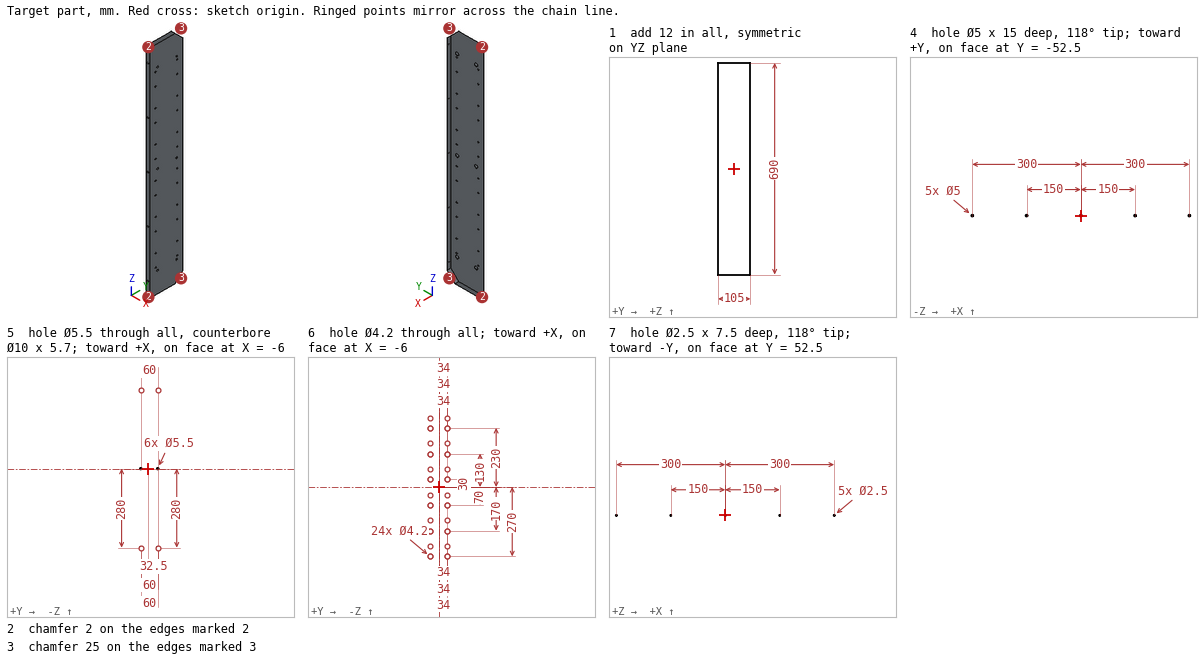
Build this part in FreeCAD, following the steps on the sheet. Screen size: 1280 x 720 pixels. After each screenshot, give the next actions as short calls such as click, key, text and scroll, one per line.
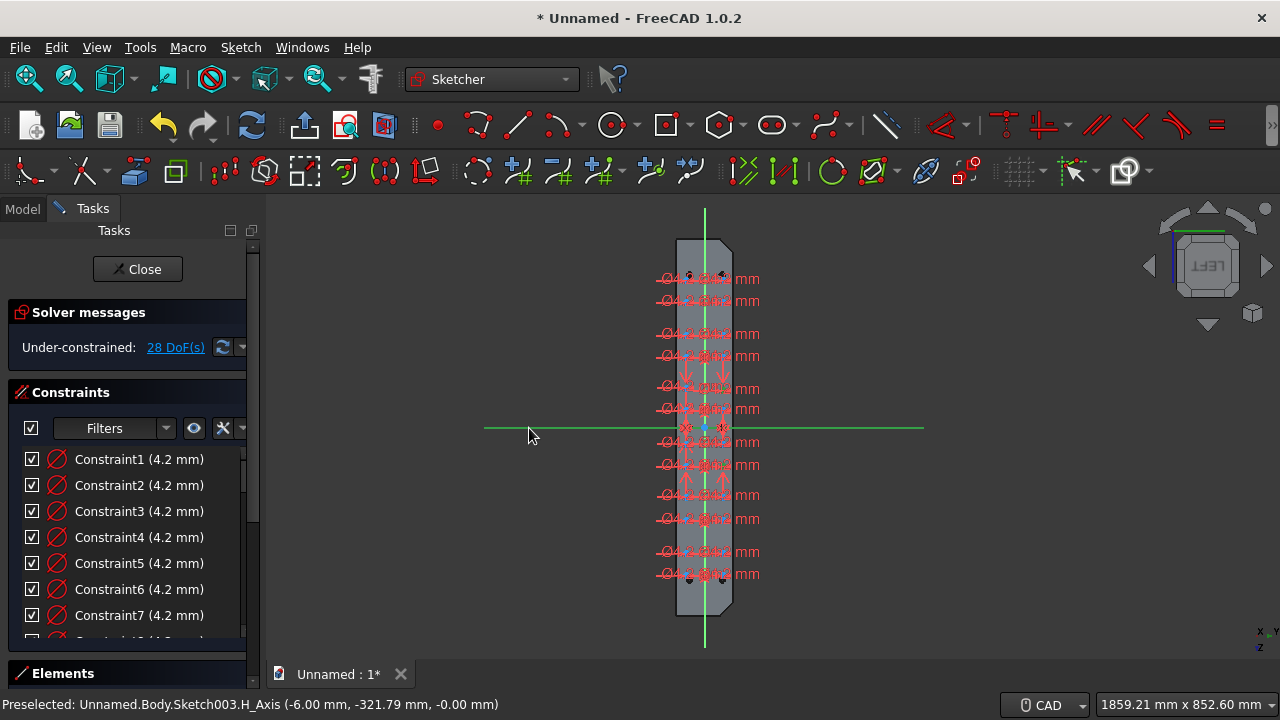
key(s)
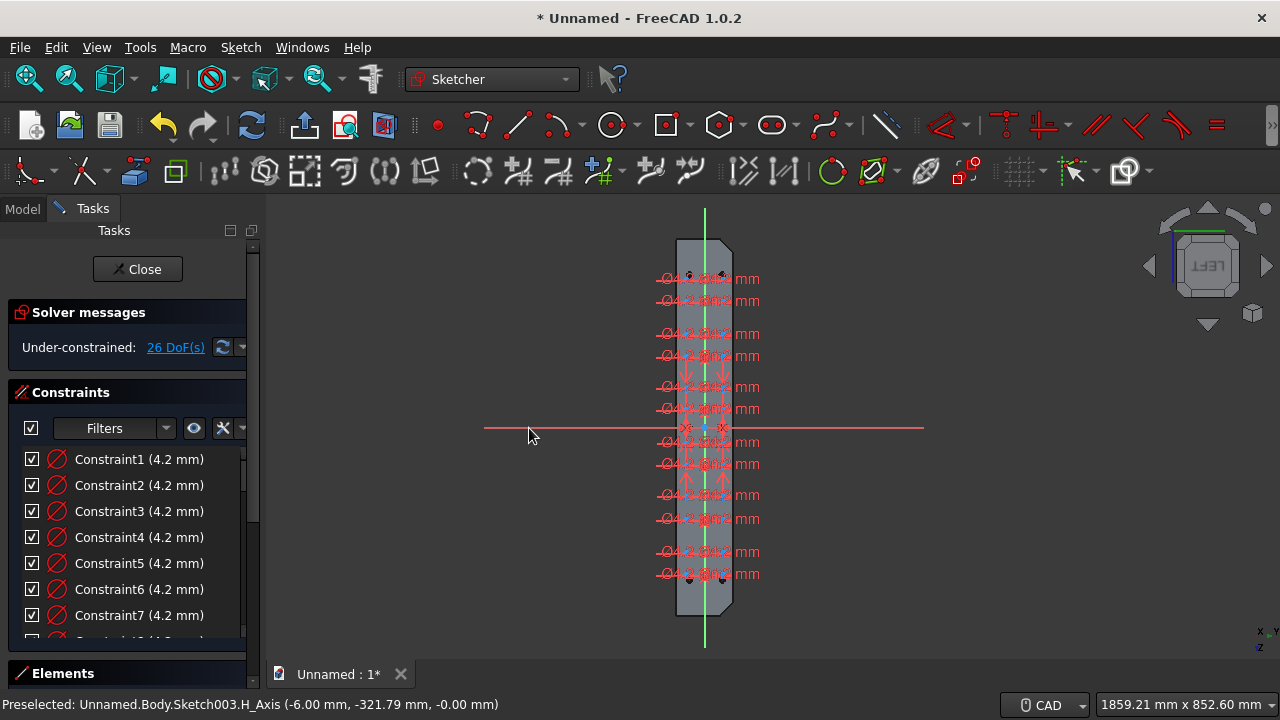
click(686, 521)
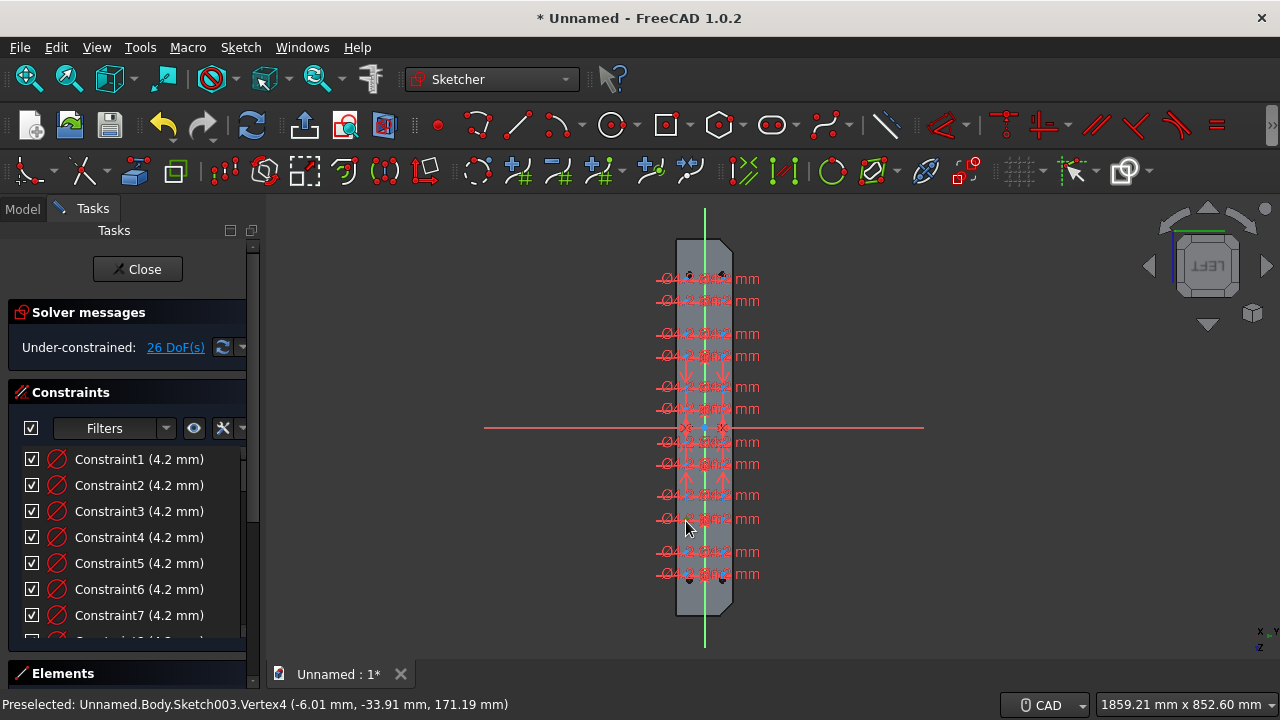
click(686, 336)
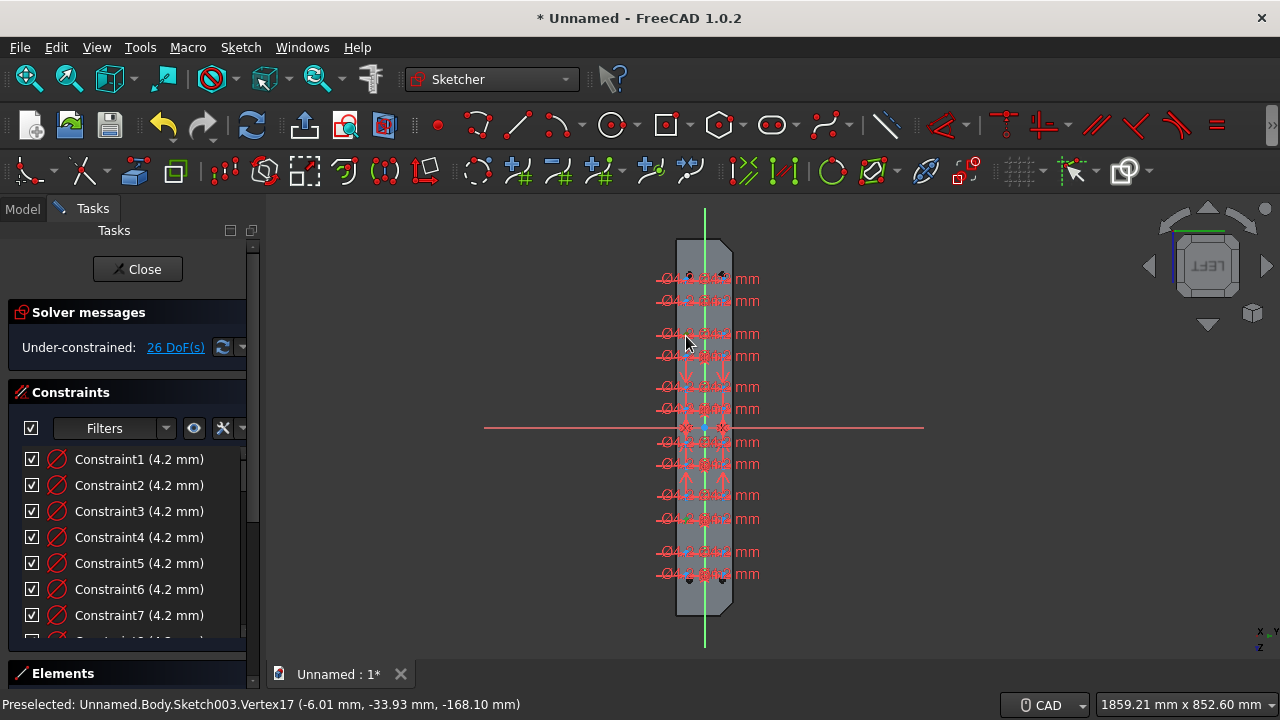
click(529, 428)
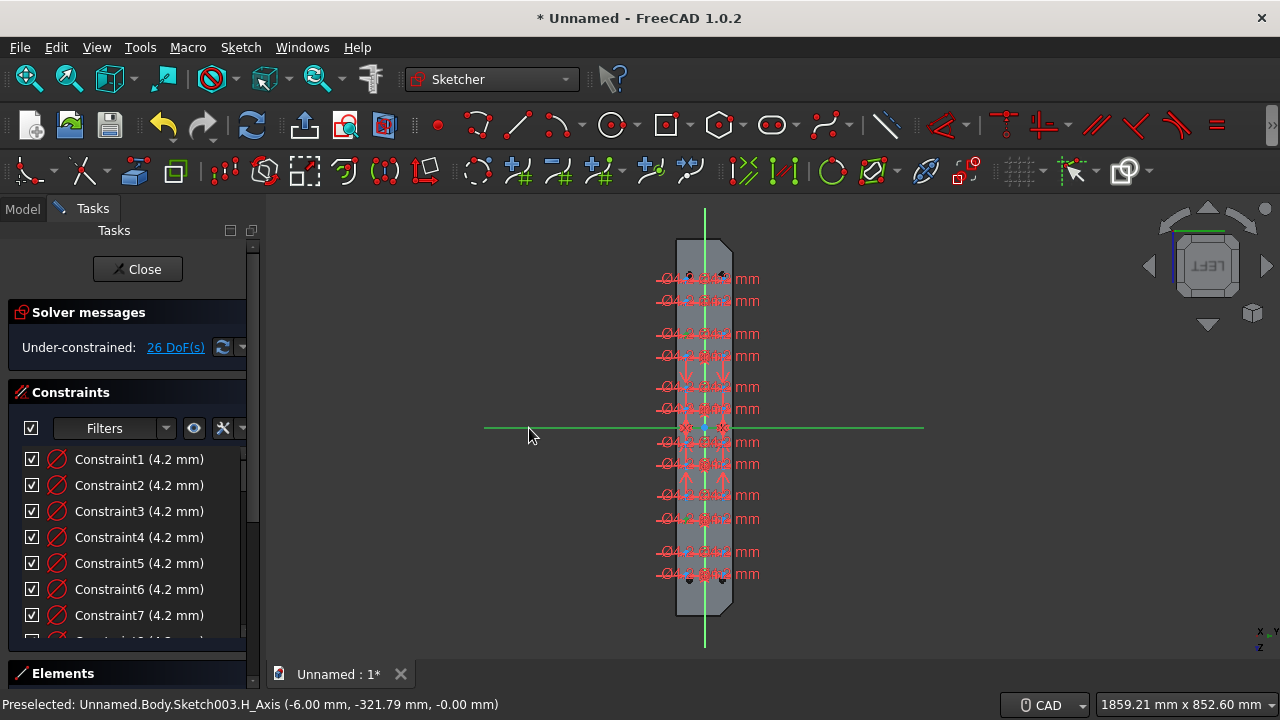
key(s)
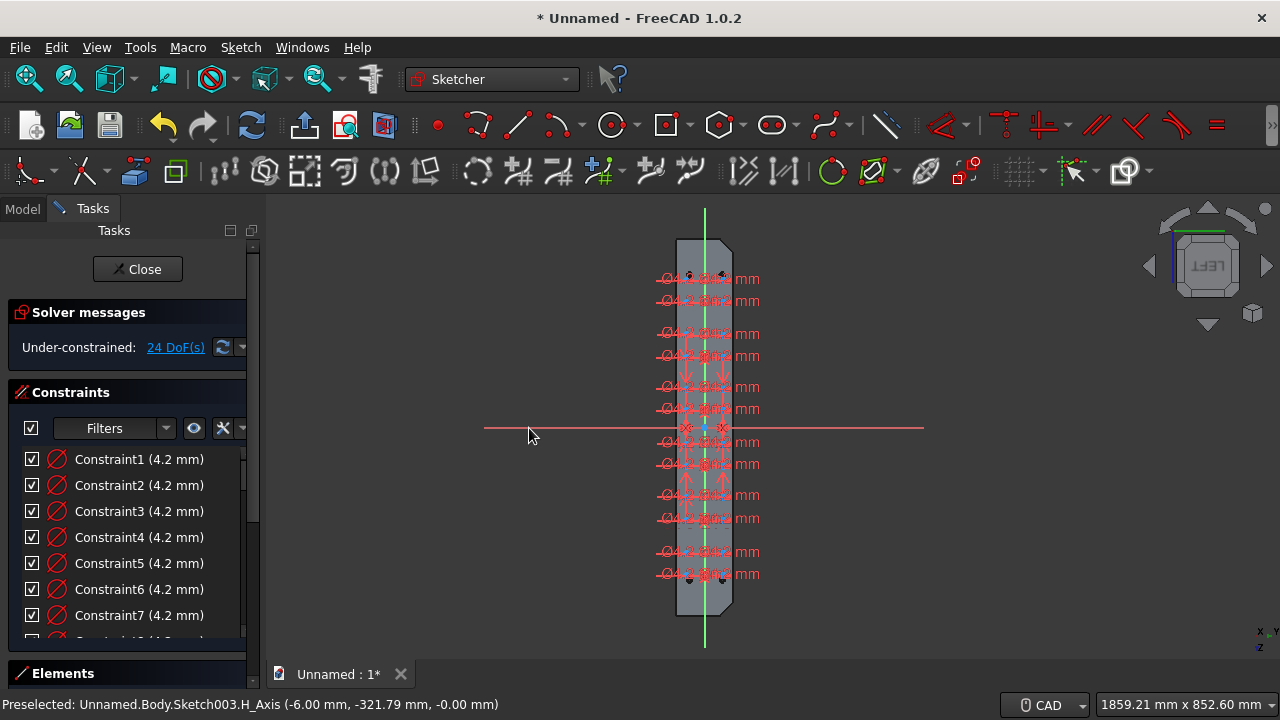
click(723, 520)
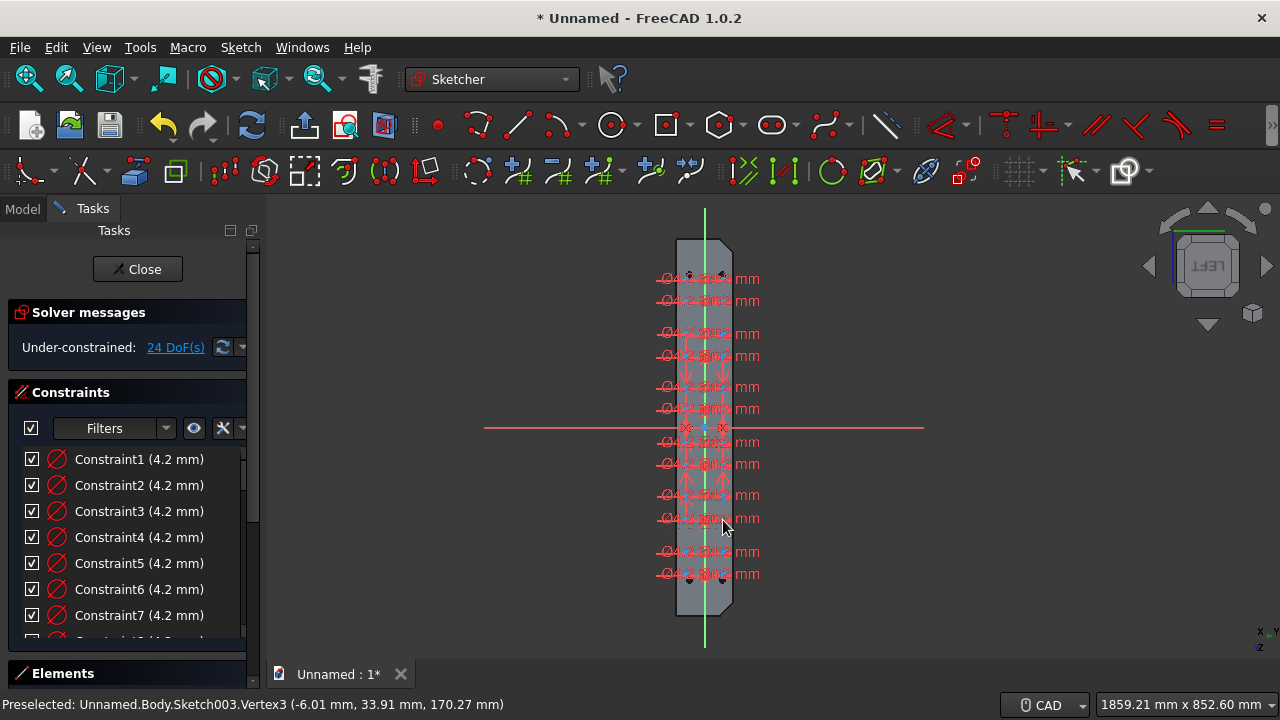
click(723, 336)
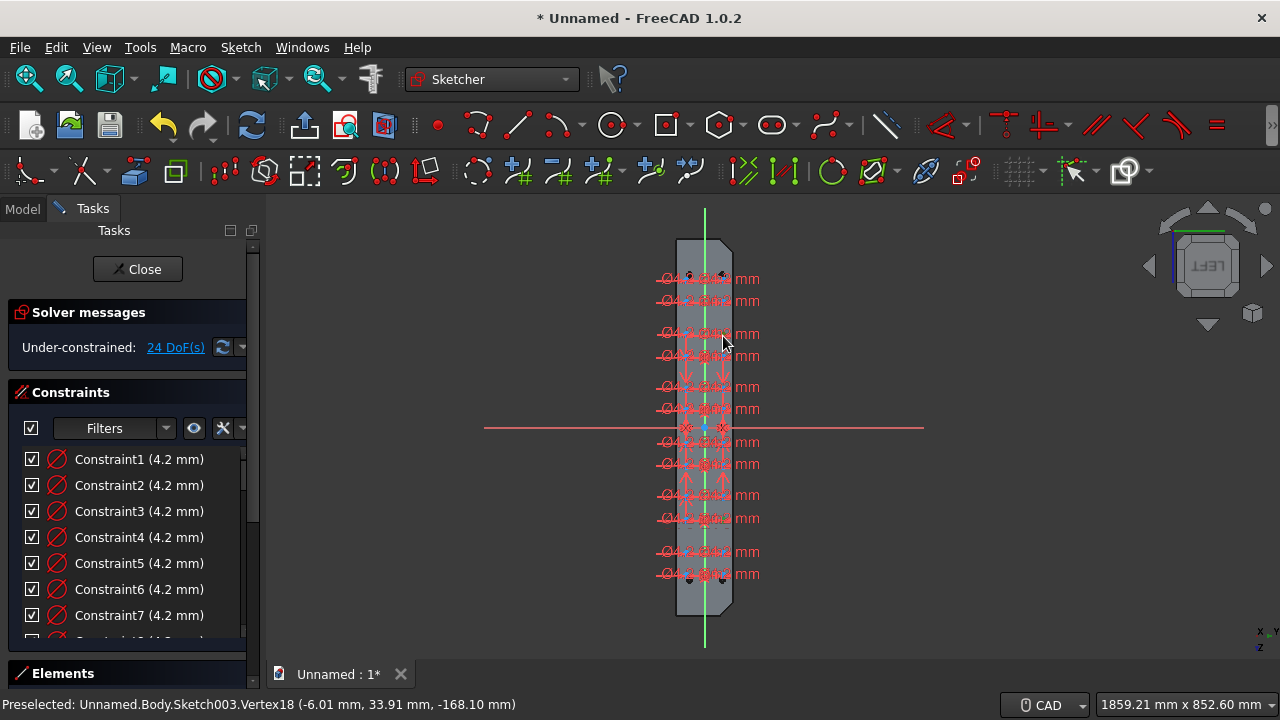
click(529, 428)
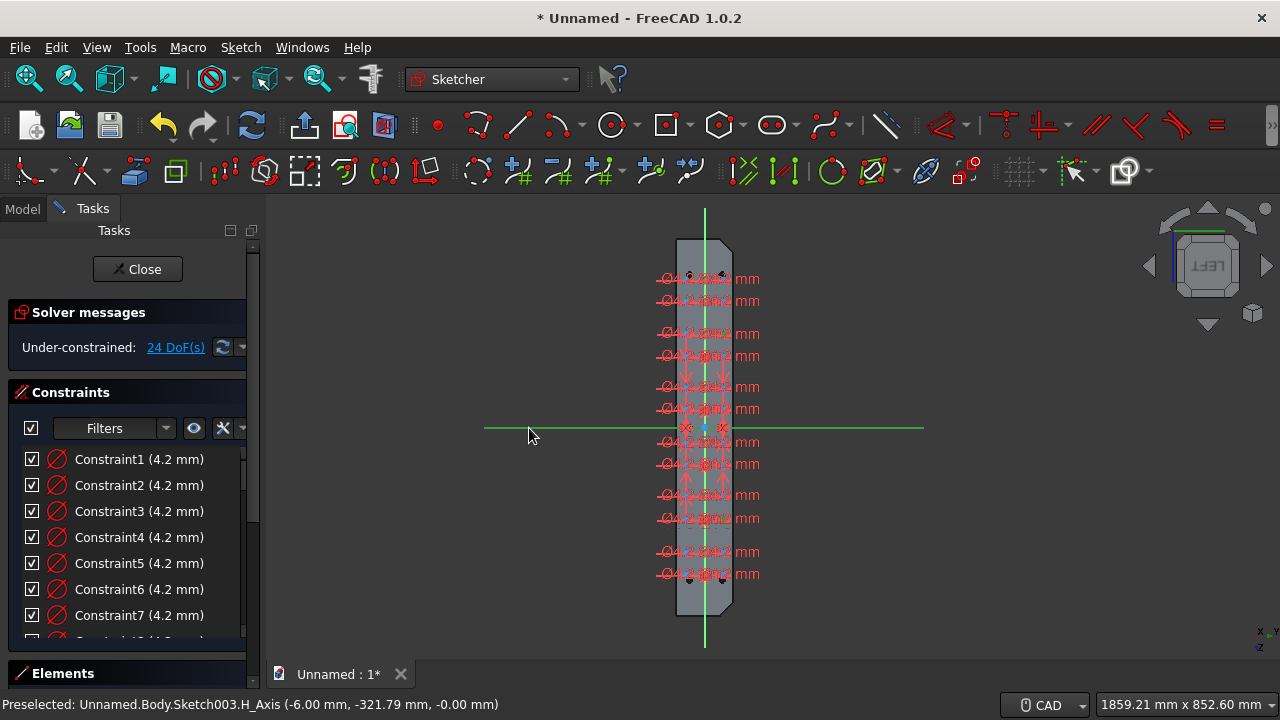
key(s)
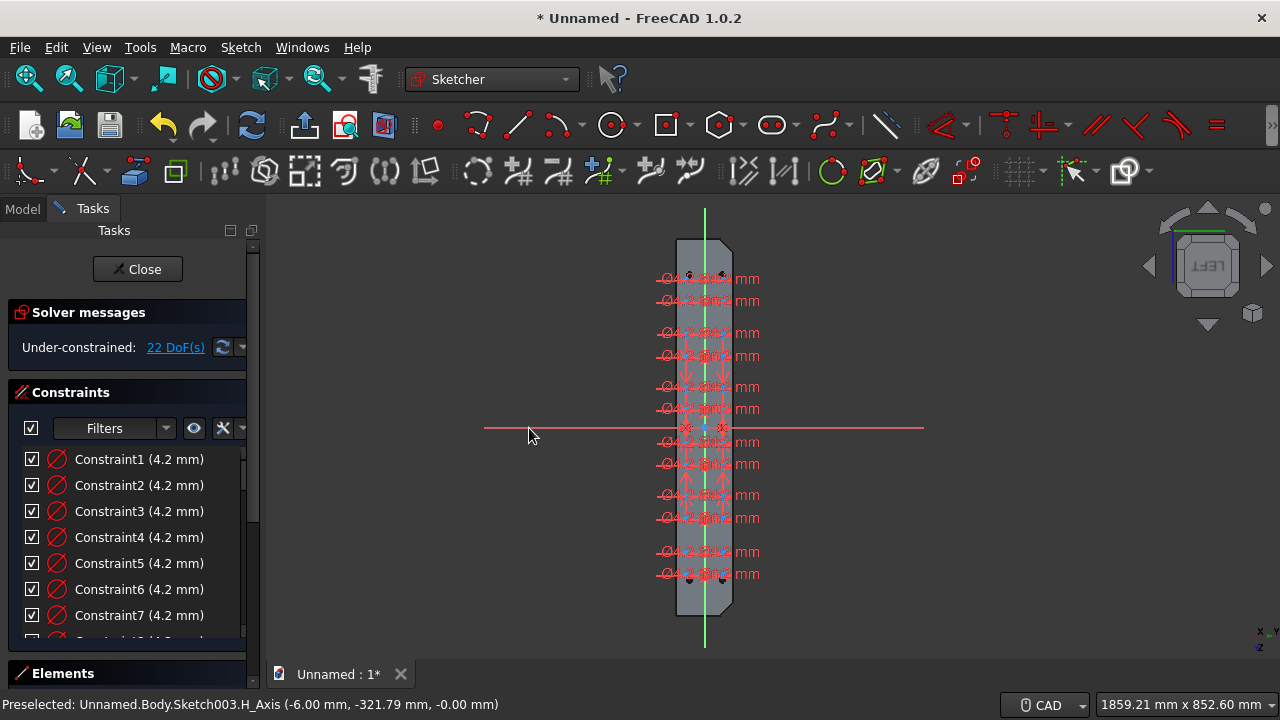
click(686, 576)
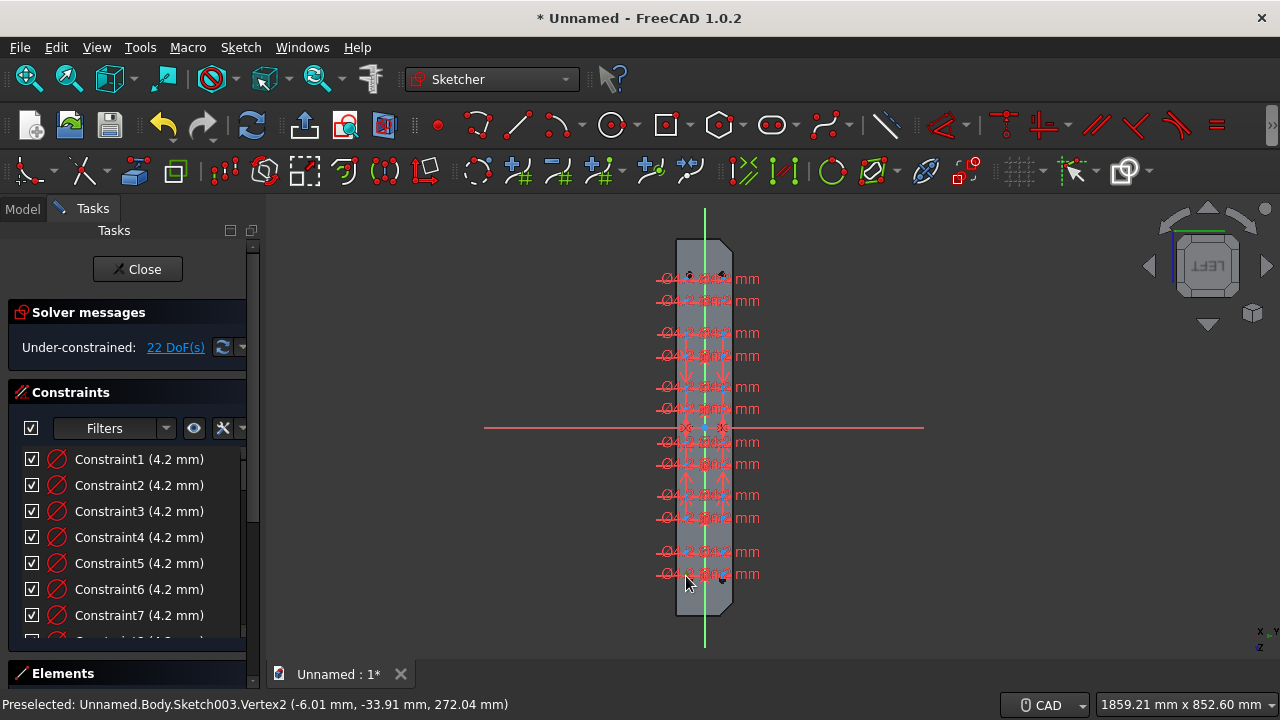
click(686, 281)